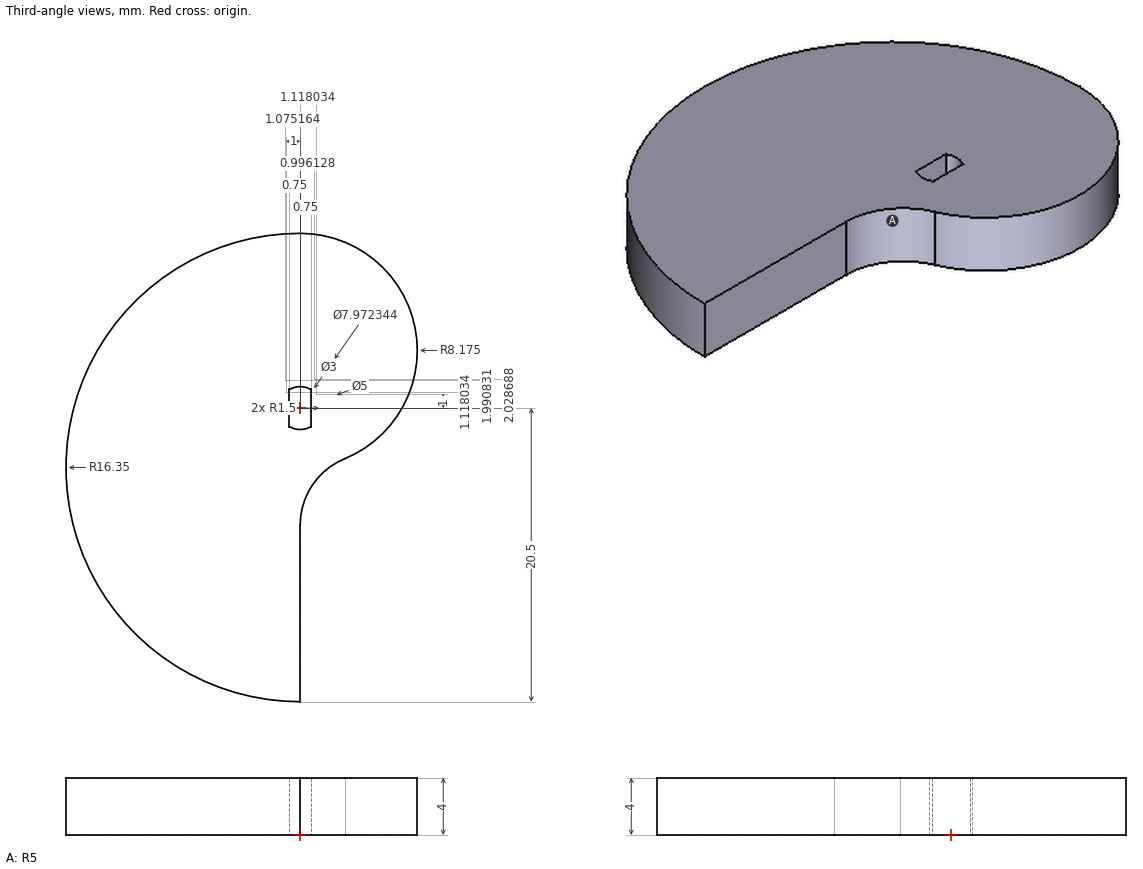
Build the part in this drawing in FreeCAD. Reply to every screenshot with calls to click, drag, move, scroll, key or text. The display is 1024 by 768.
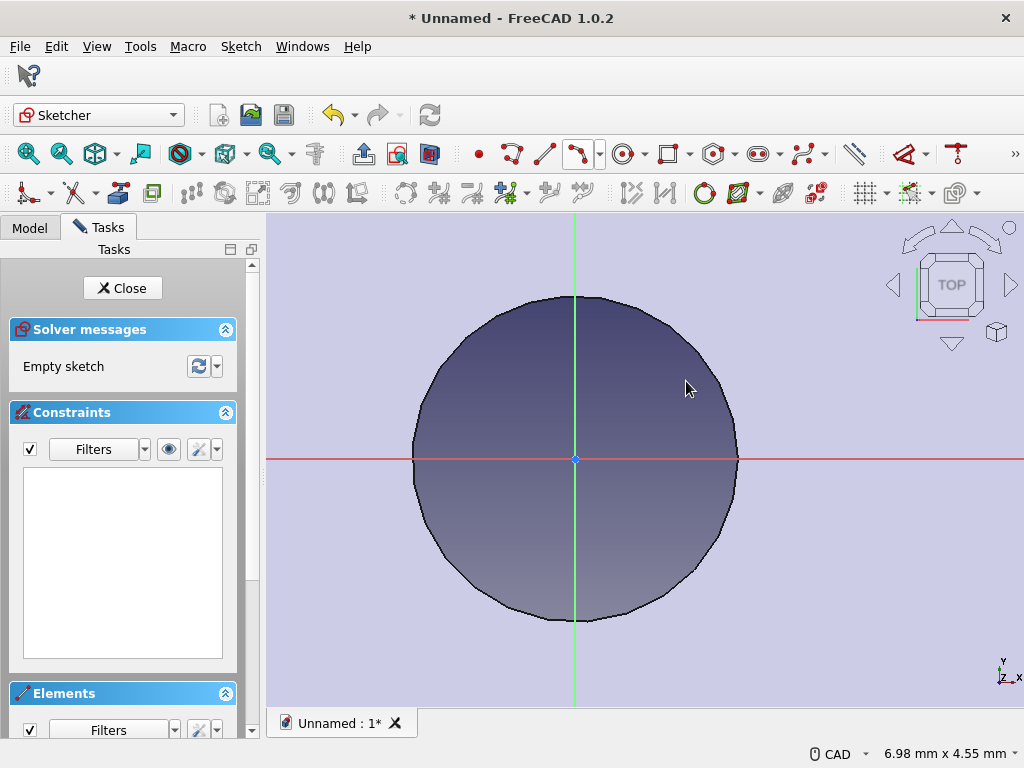
click(545, 154)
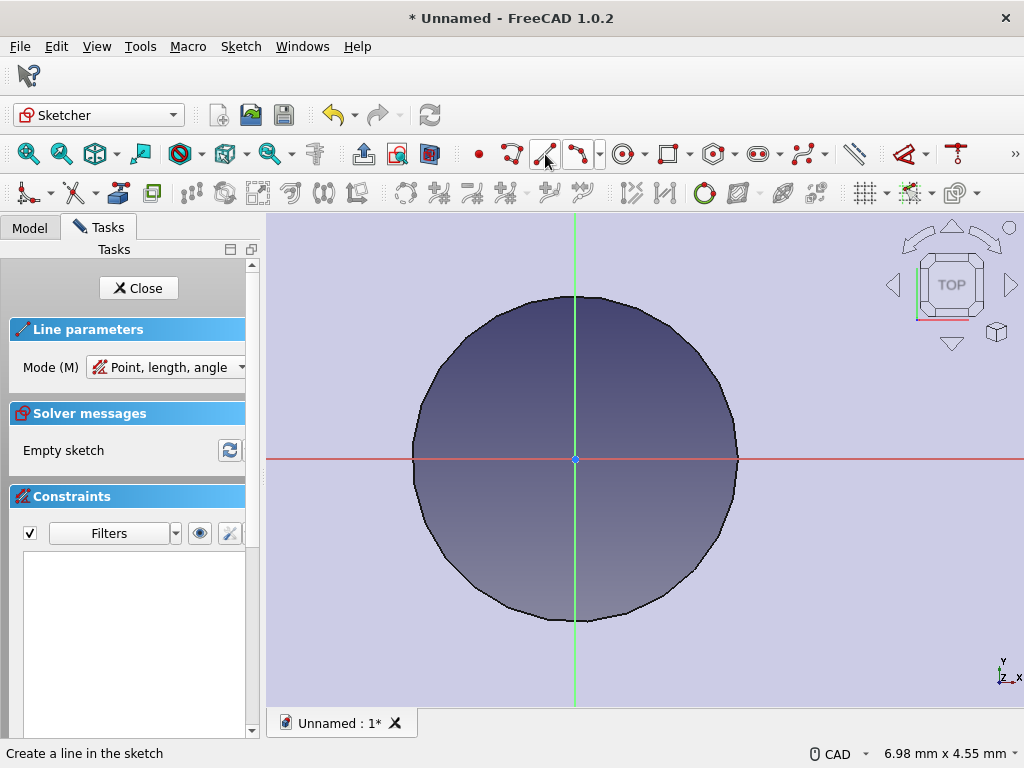
click(657, 318)
click(657, 600)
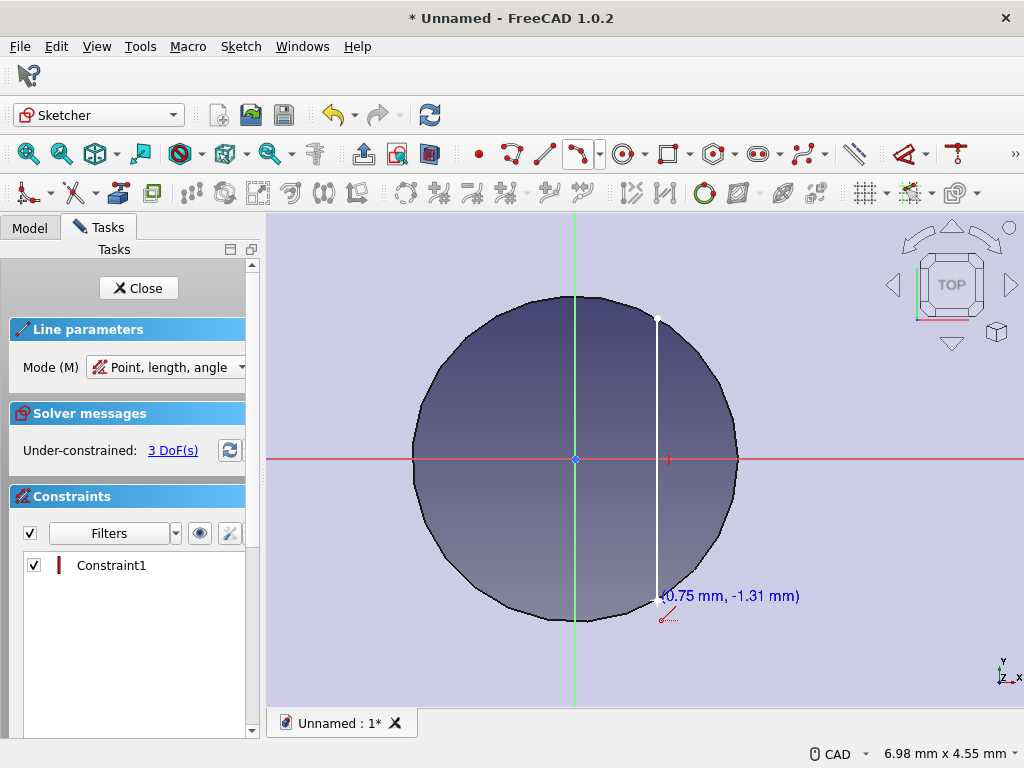
click(578, 154)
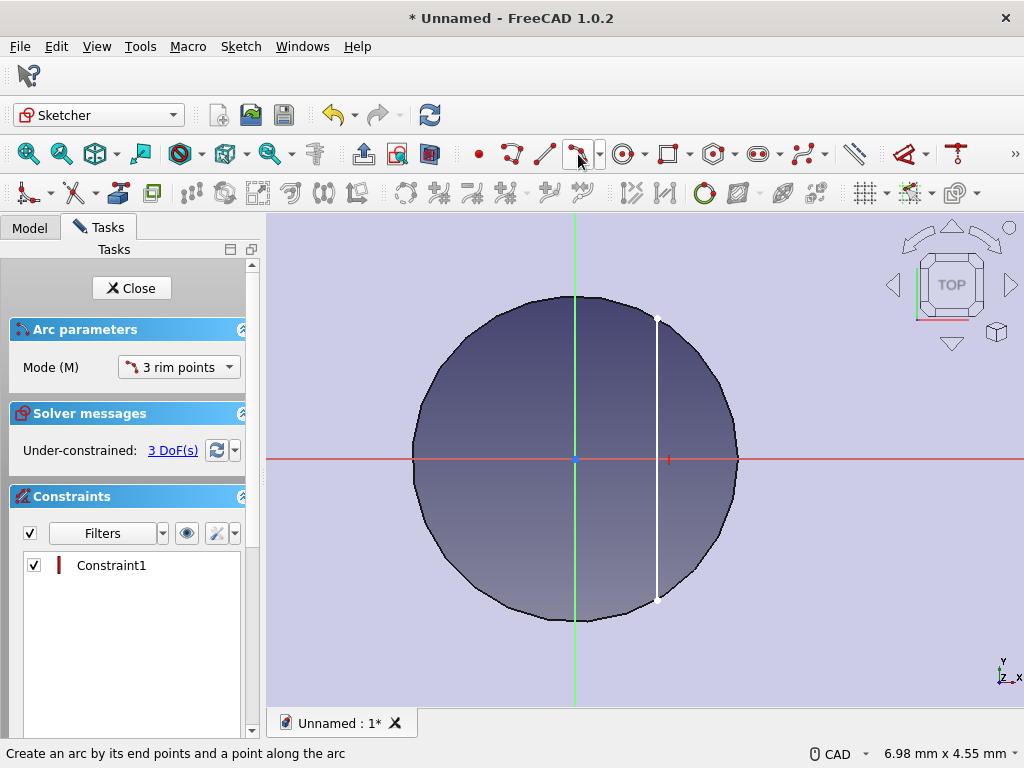
click(657, 601)
click(657, 319)
click(734, 493)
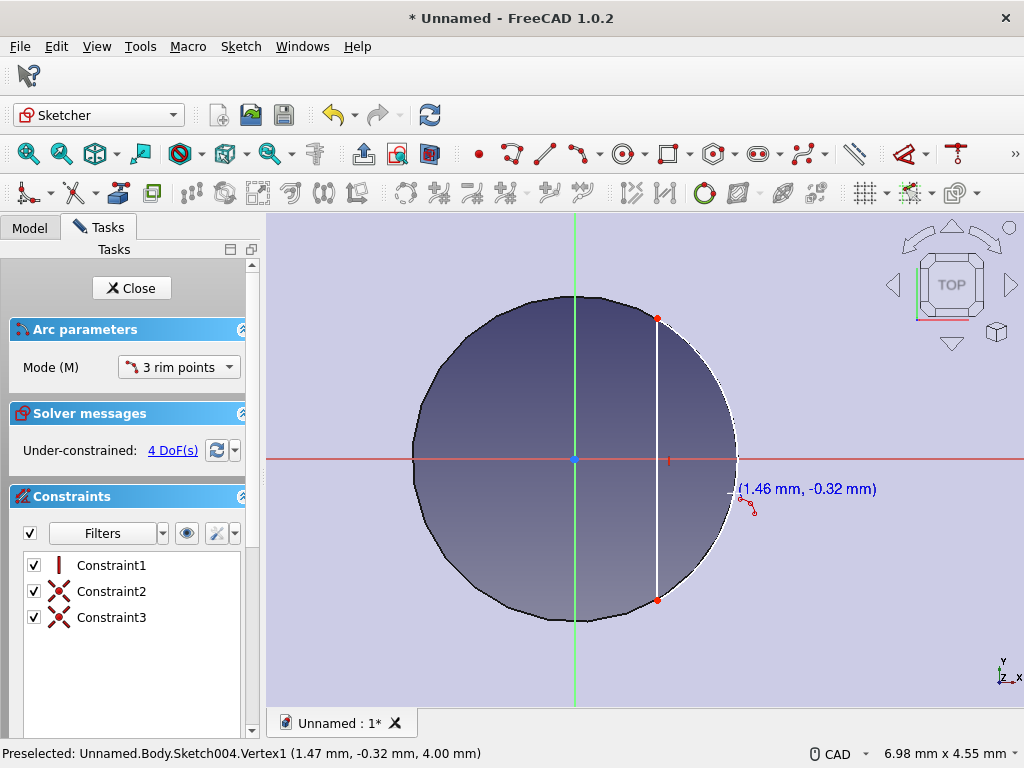
key(g)
key(l)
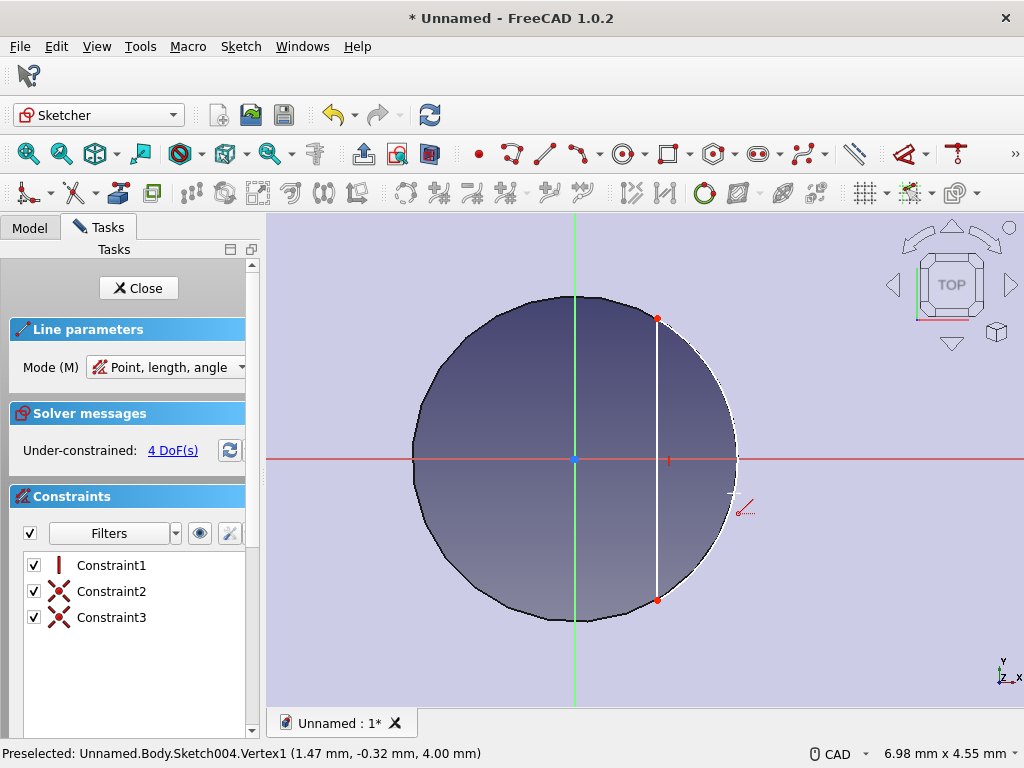
click(494, 600)
click(494, 318)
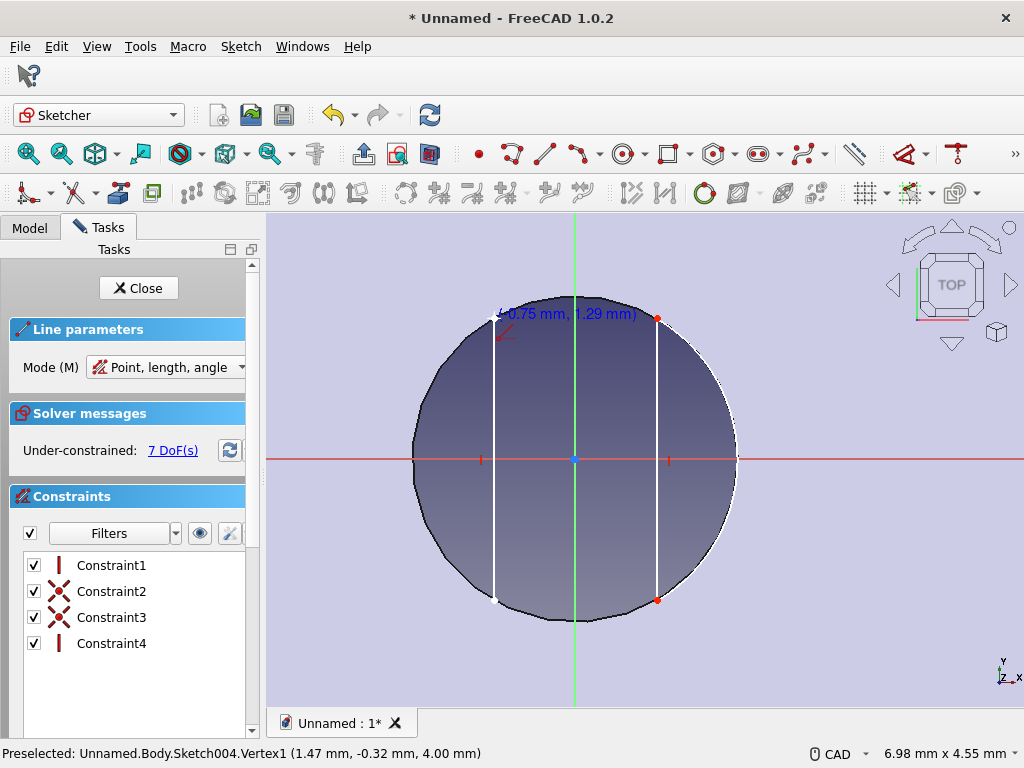
key(g)
key(3)
key(a)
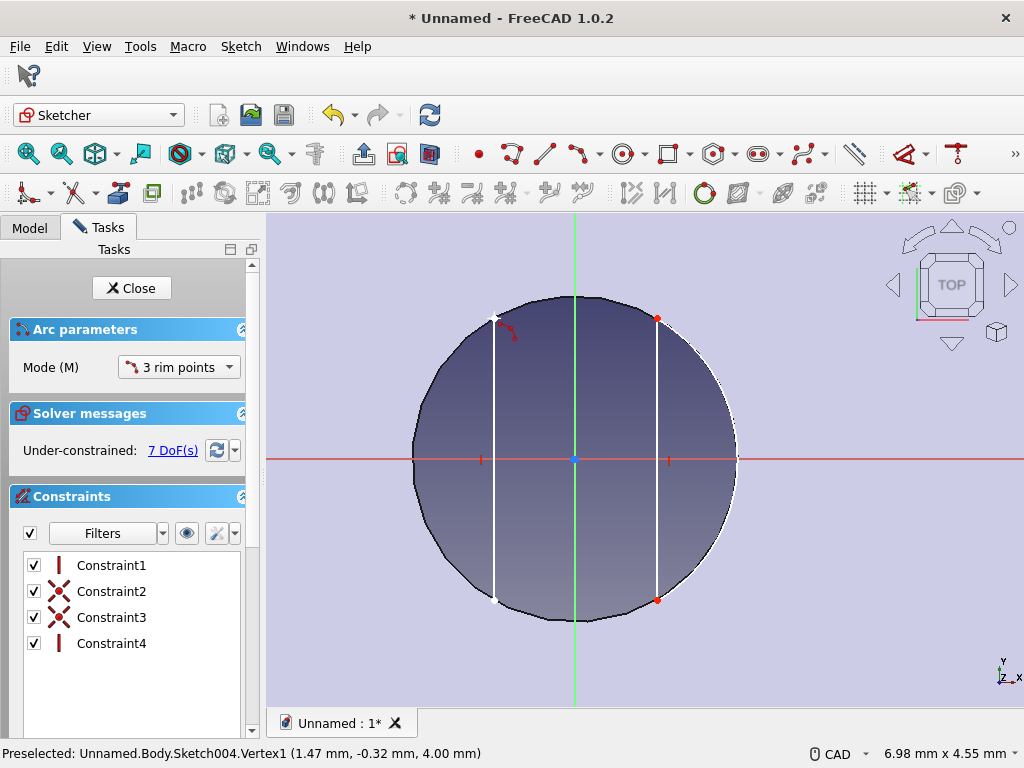
click(494, 319)
click(494, 601)
click(416, 425)
key(Escape)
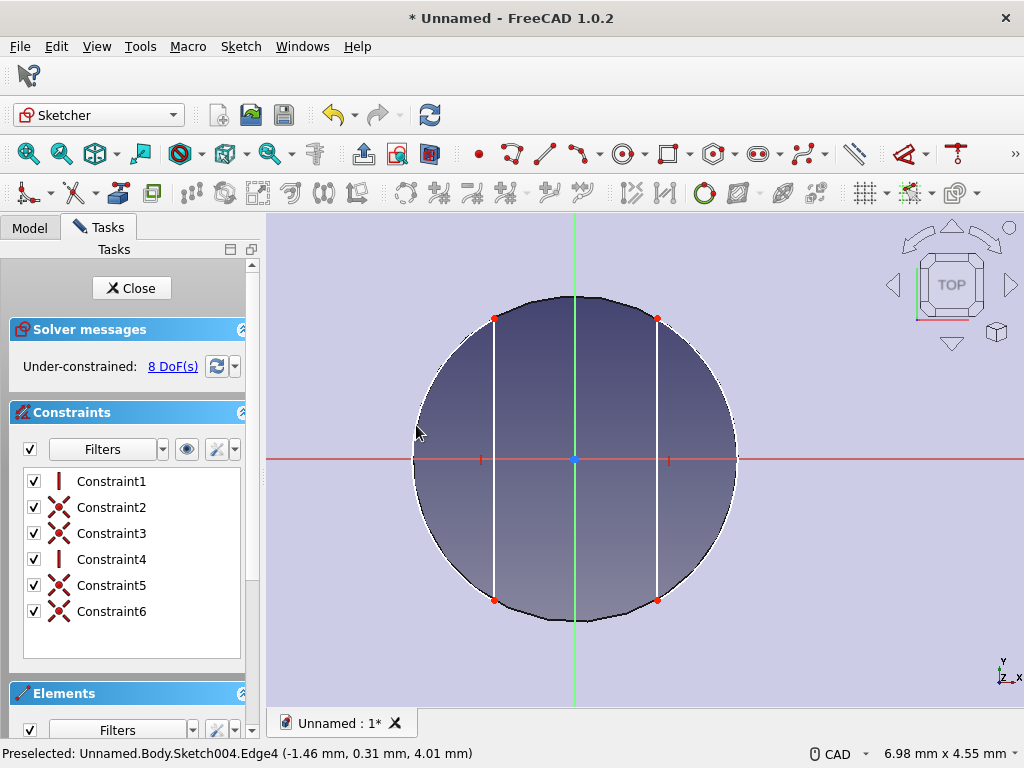
click(724, 526)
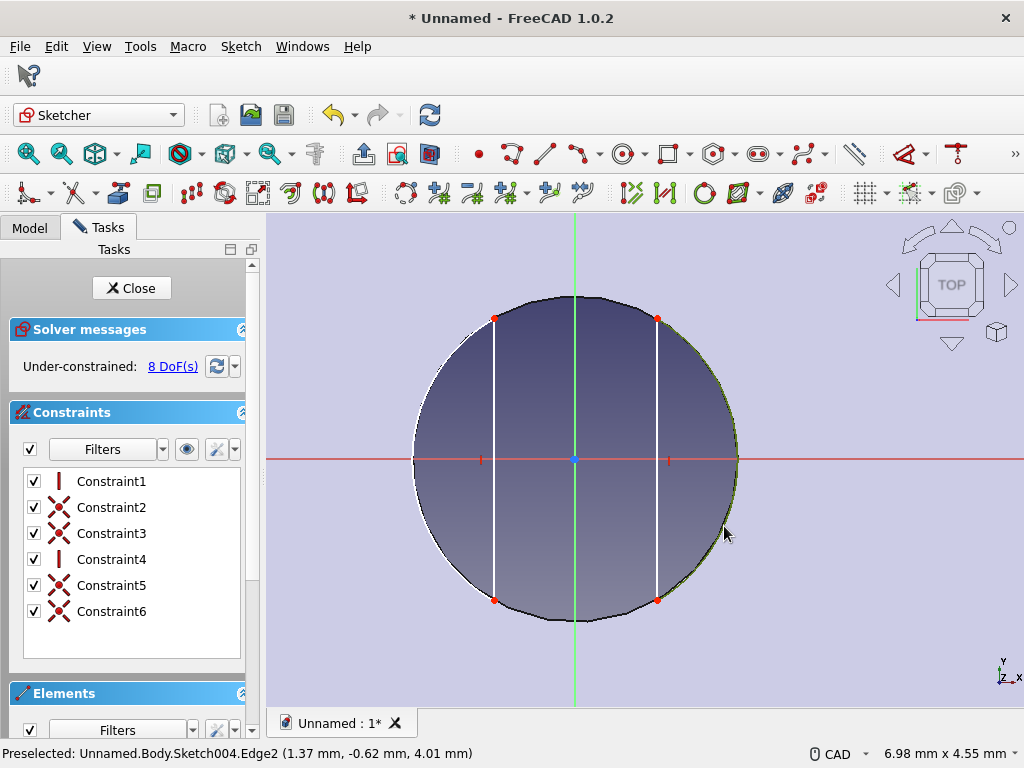
click(427, 394)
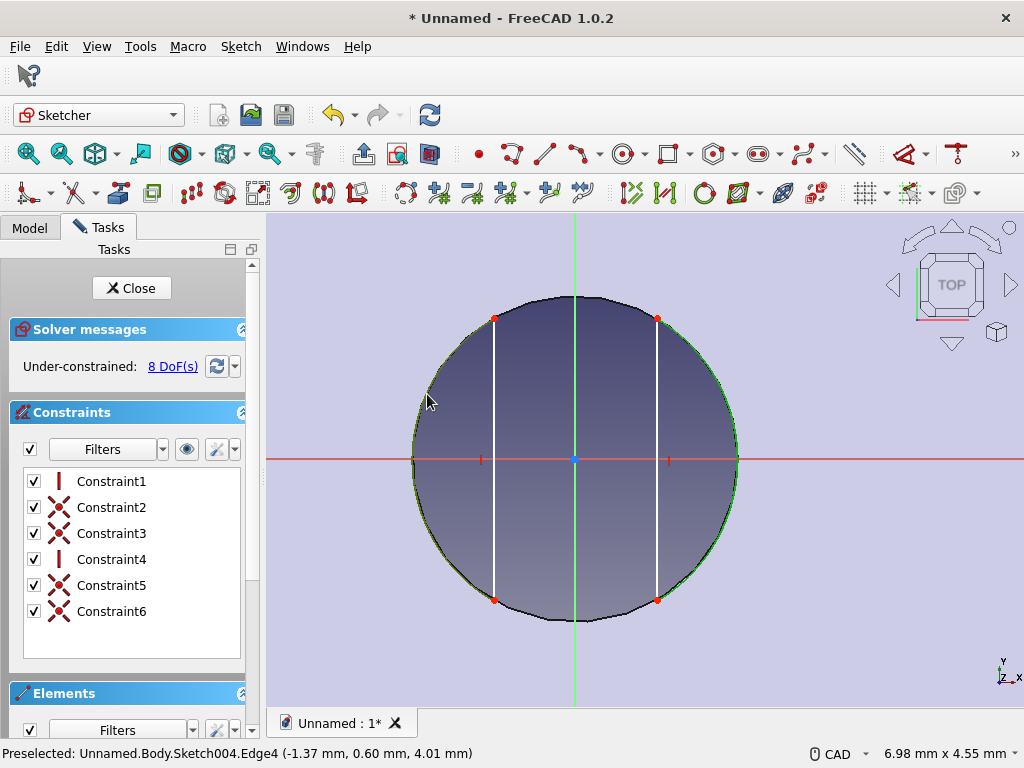
click(956, 154)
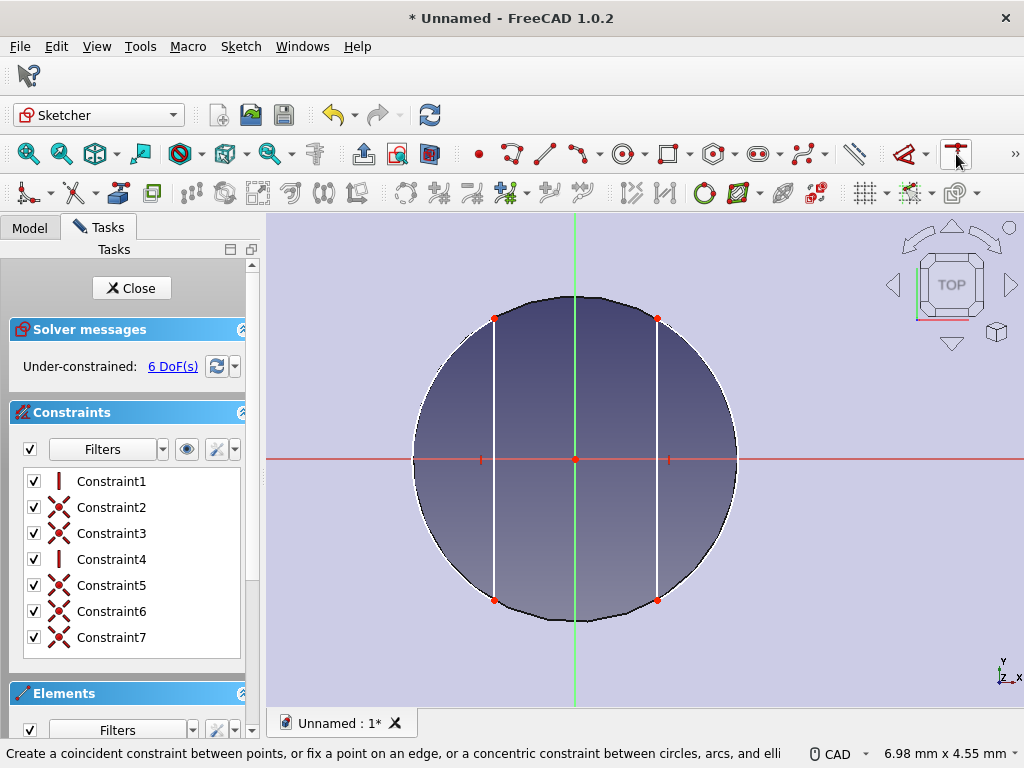
drag(565, 449, 585, 470)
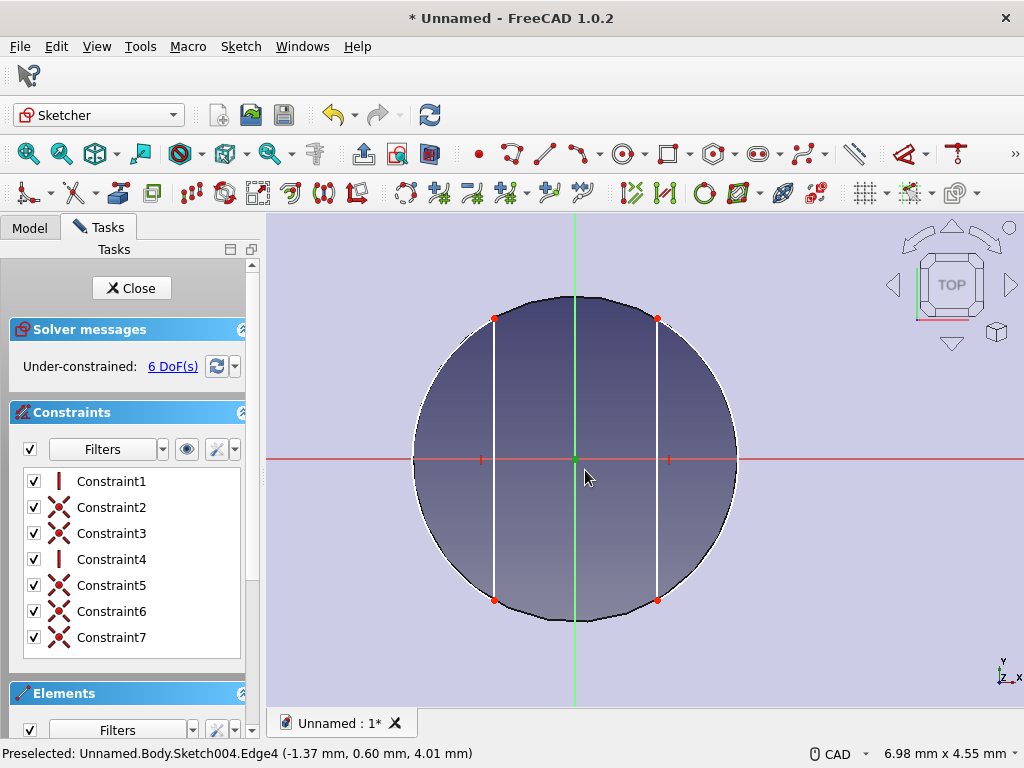
key(c)